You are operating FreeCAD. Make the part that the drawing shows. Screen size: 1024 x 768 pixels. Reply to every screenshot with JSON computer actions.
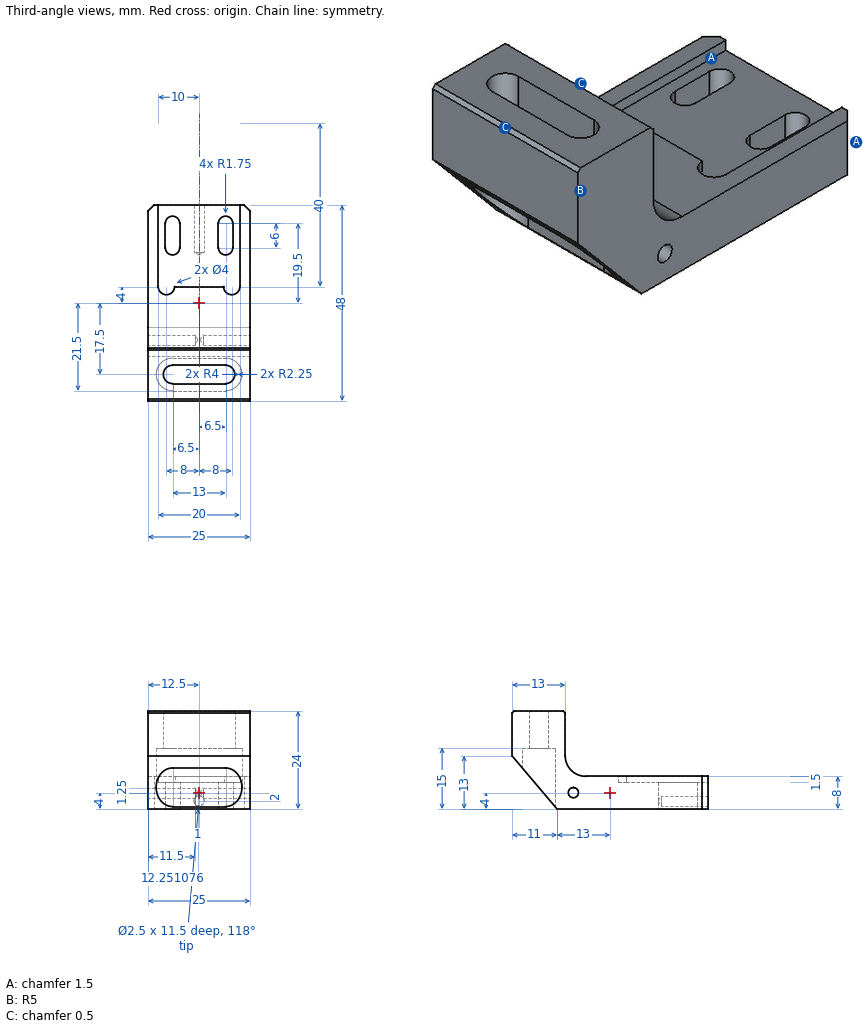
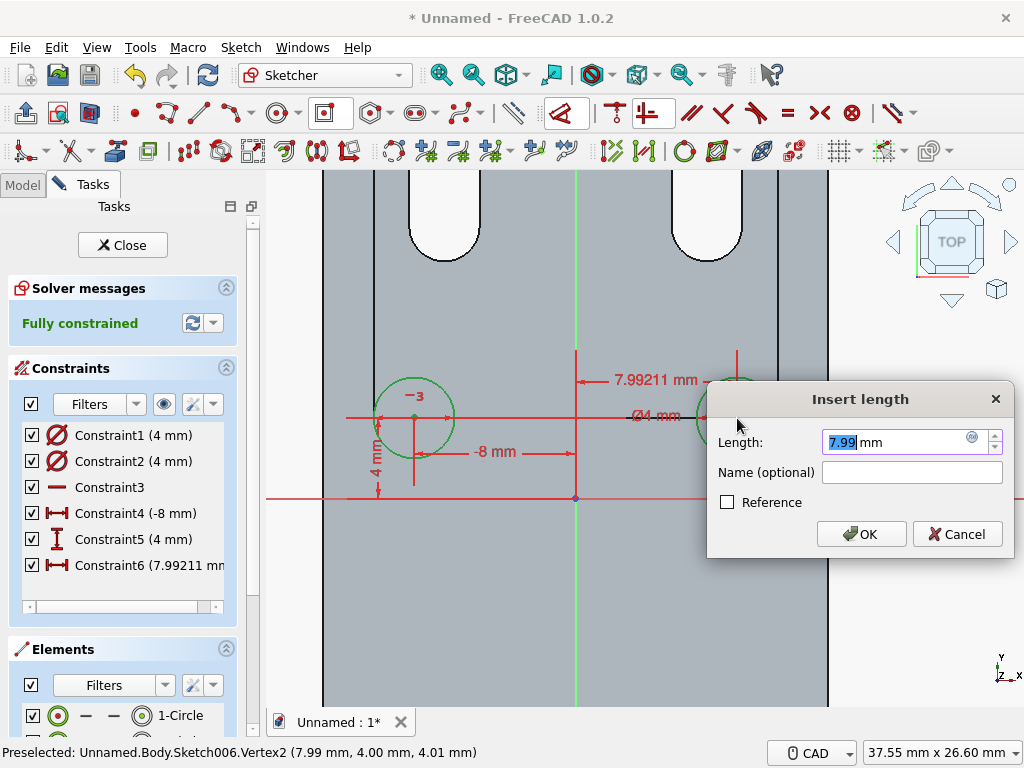
{"action": "type", "text": "8"}
{"action": "key", "text": "Return"}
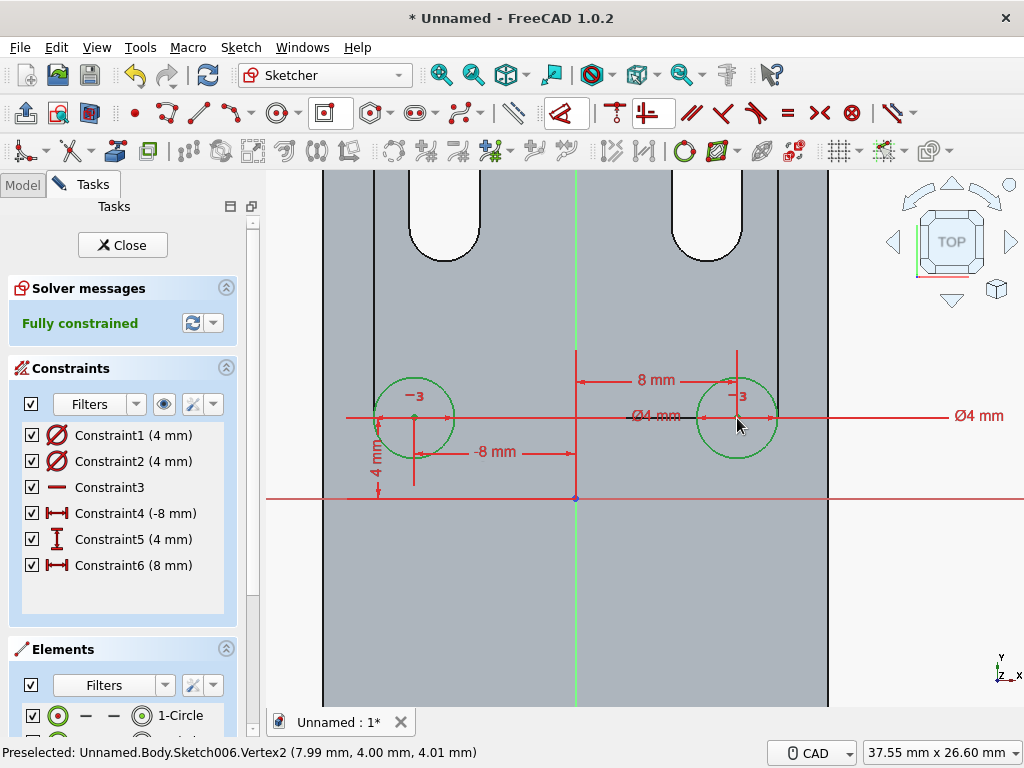
{"action": "left_click", "coordinate": [123, 245]}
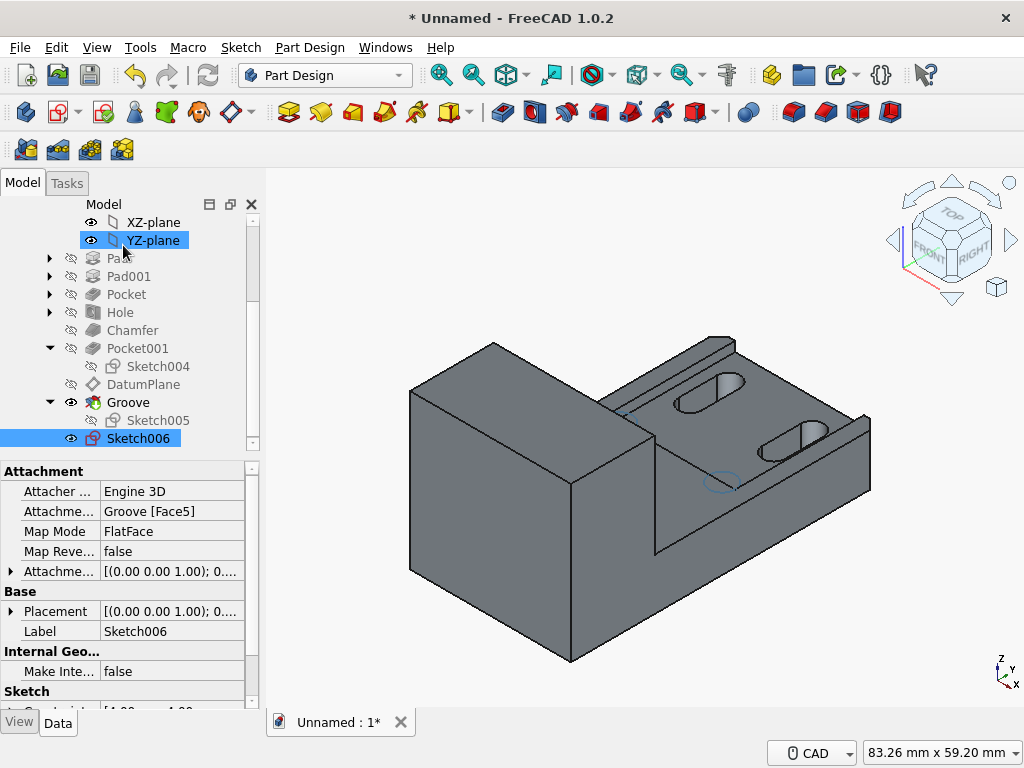
{"action": "left_click", "coordinate": [504, 112]}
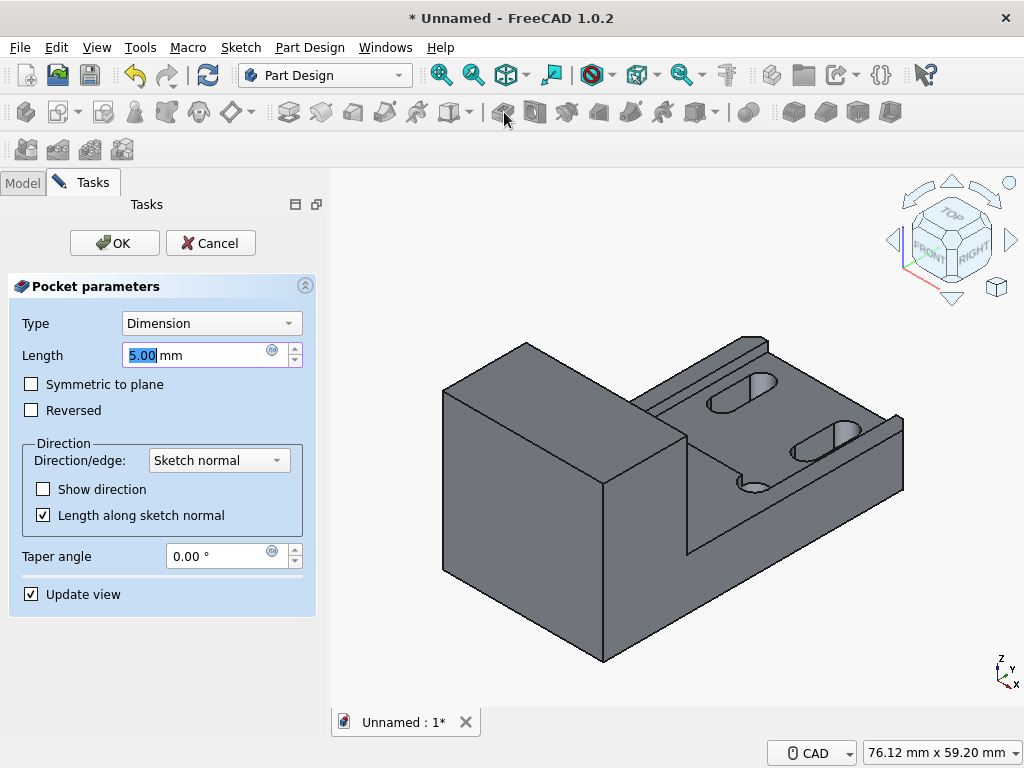
{"action": "type", "text": "1.5"}
{"action": "key", "text": "Tab"}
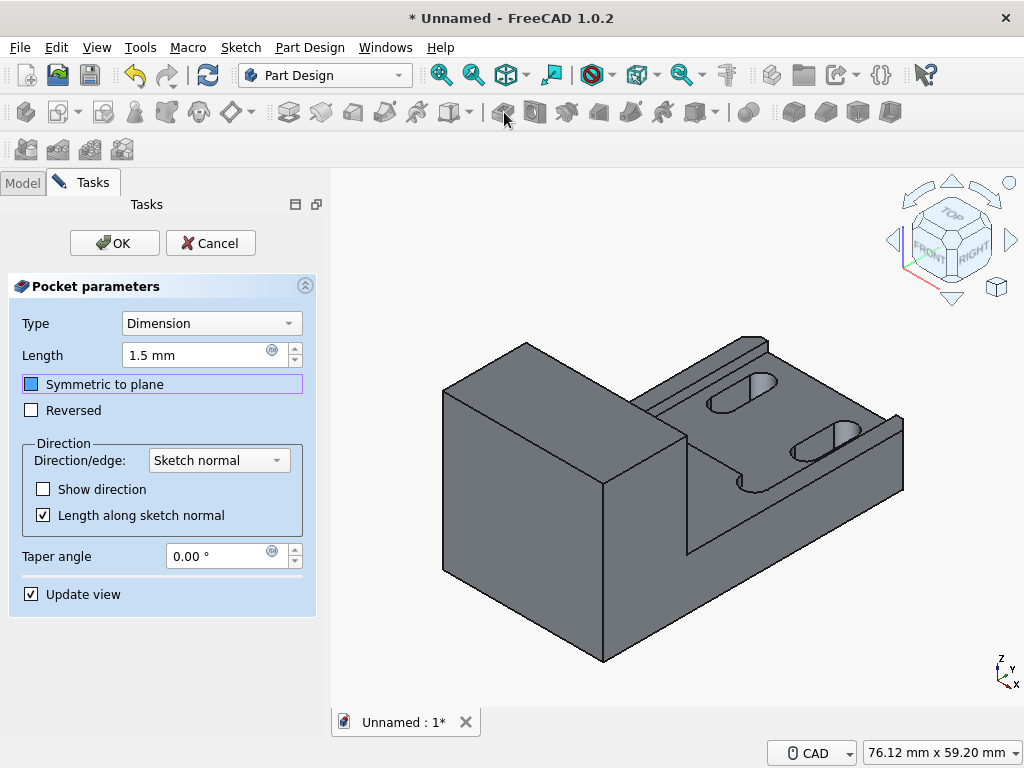
{"action": "left_click", "coordinate": [115, 243]}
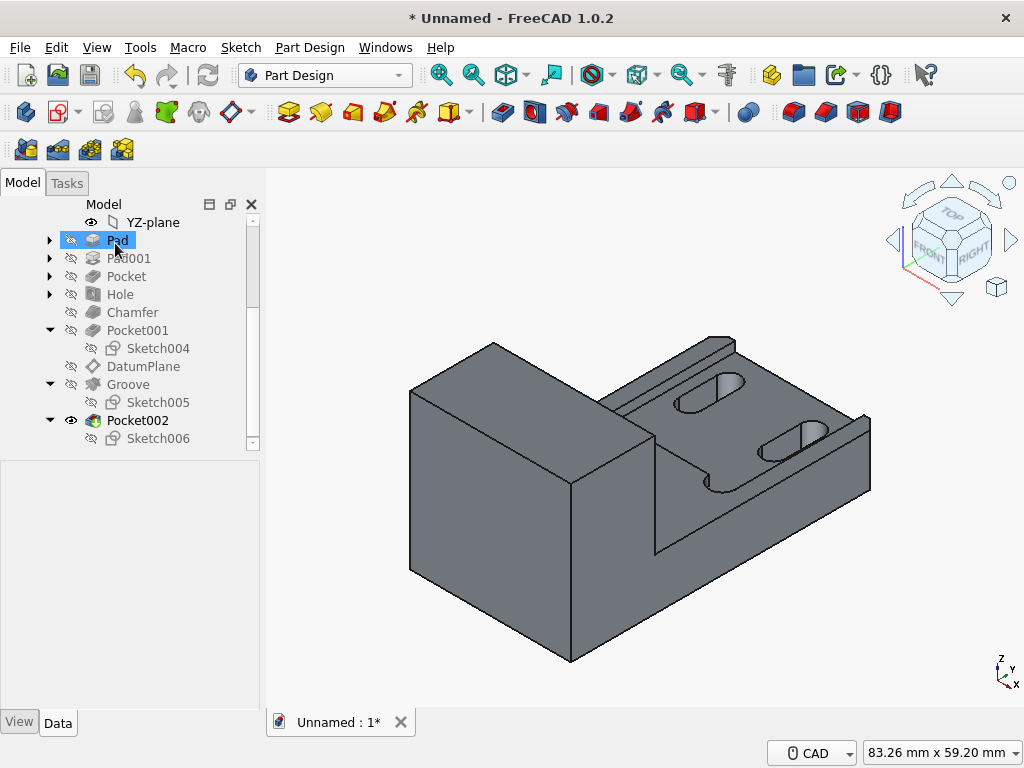
{"action": "key", "text": "5"}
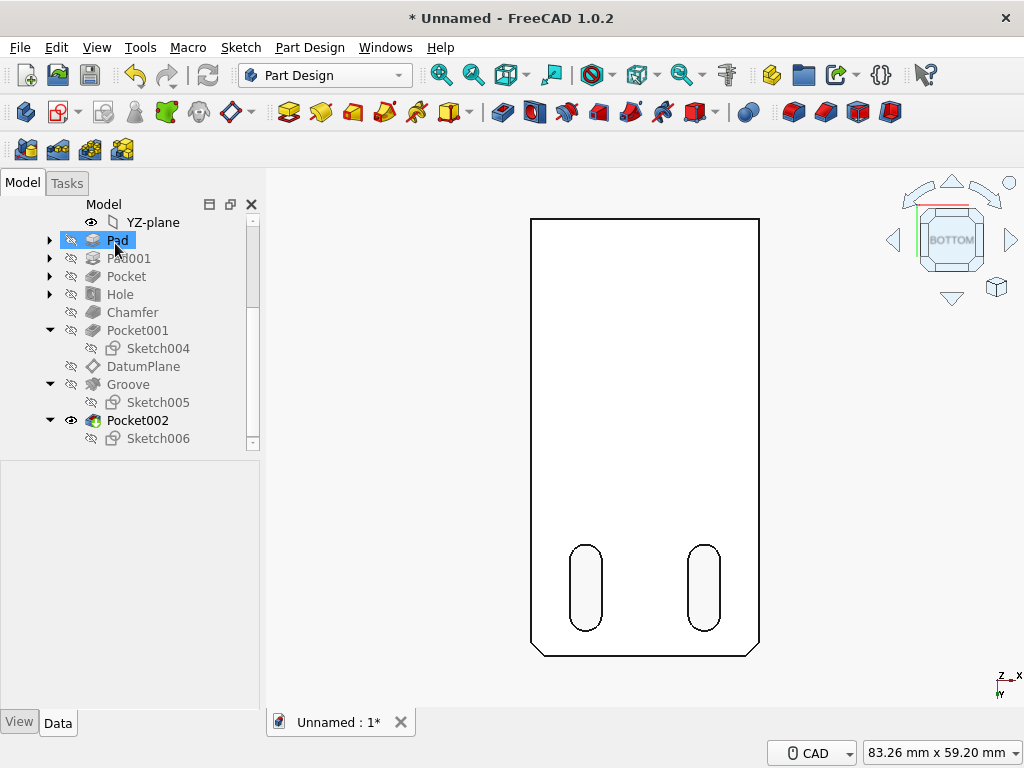
{"action": "left_click", "coordinate": [645, 437]}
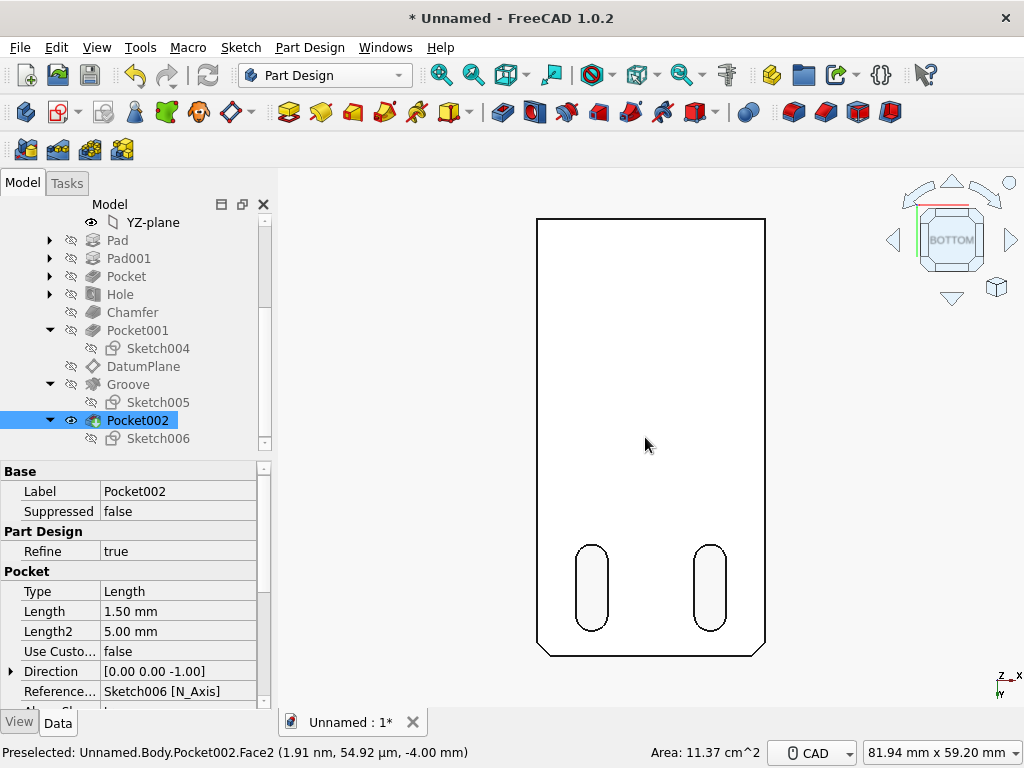
{"action": "left_click", "coordinate": [58, 112]}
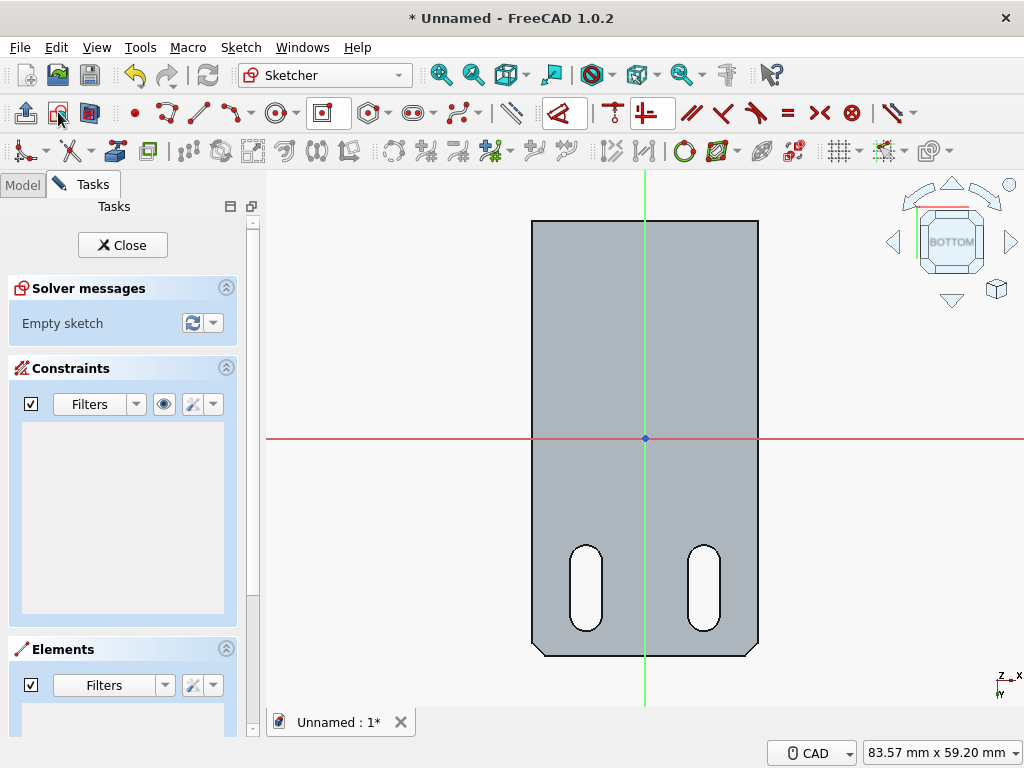
{"action": "scroll", "coordinate": [728, 240], "scroll_direction": "up", "scroll_amount": 3}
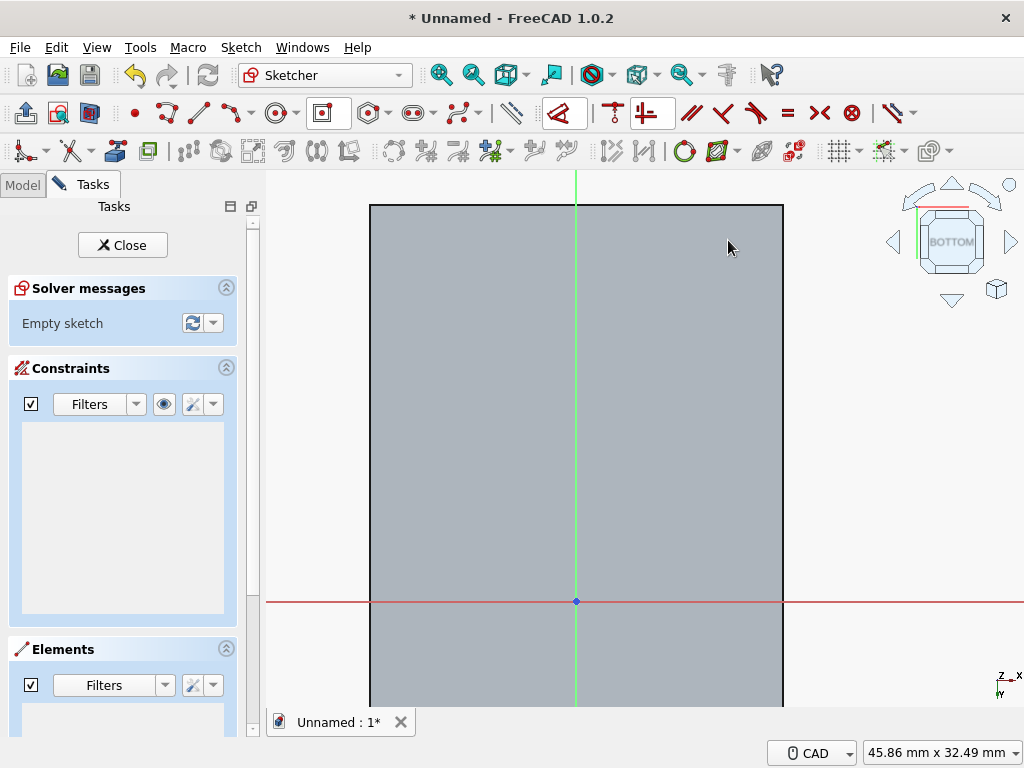
{"action": "left_click", "coordinate": [414, 114]}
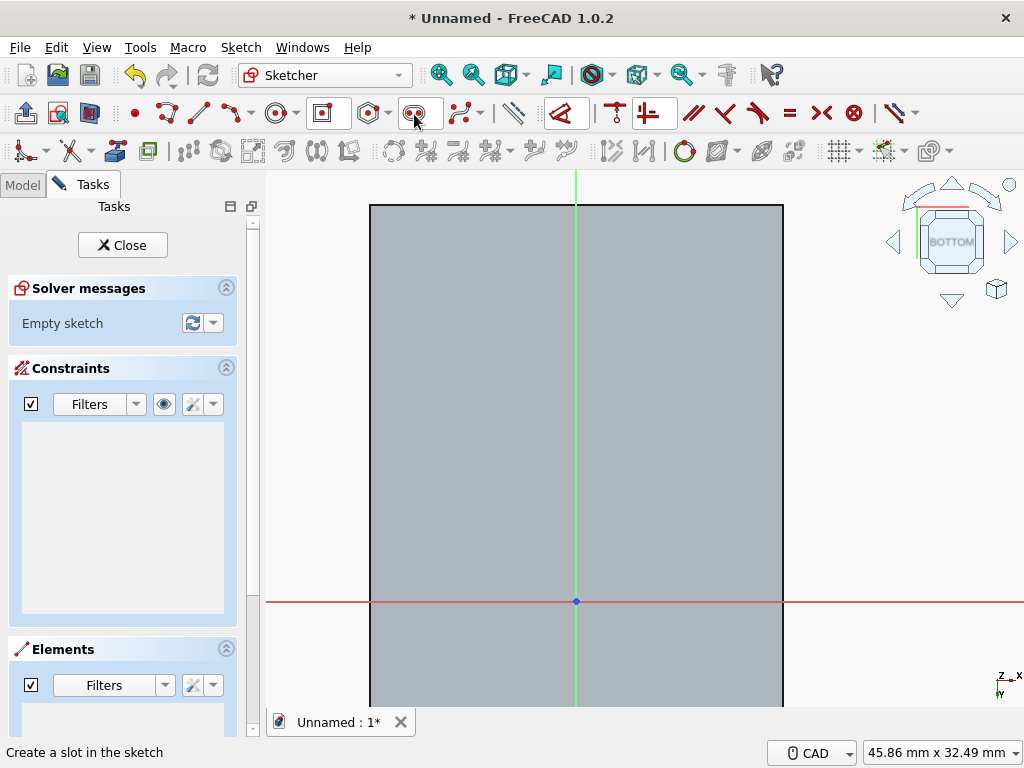
{"action": "left_click", "coordinate": [469, 312]}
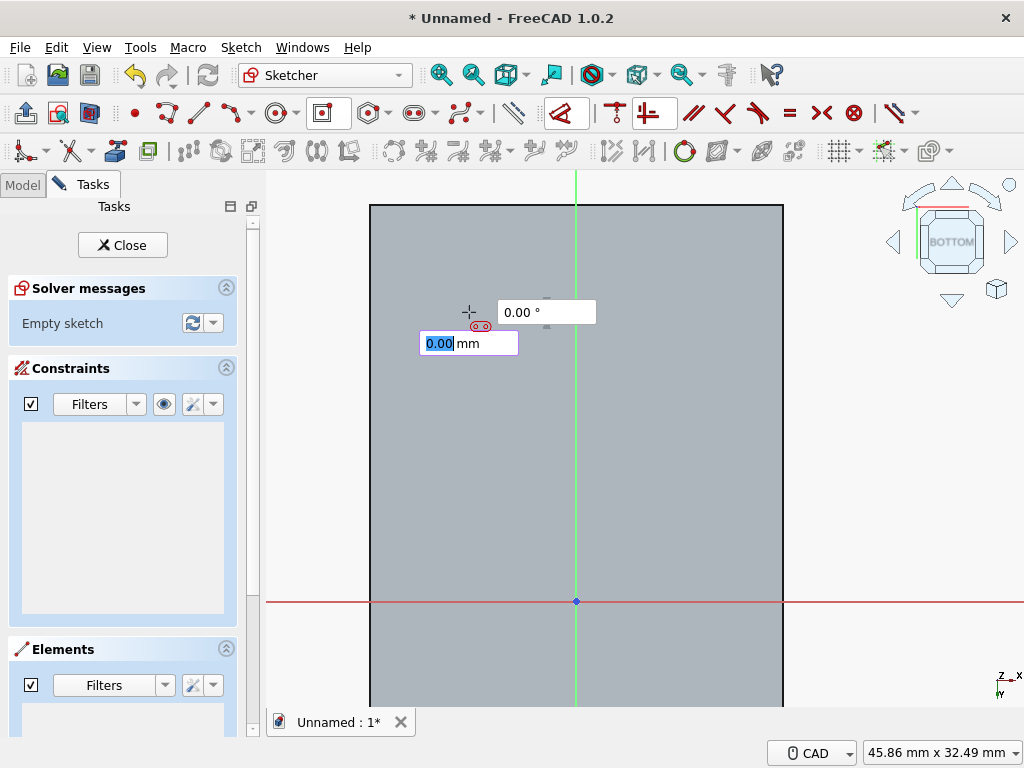
{"action": "left_click", "coordinate": [684, 312]}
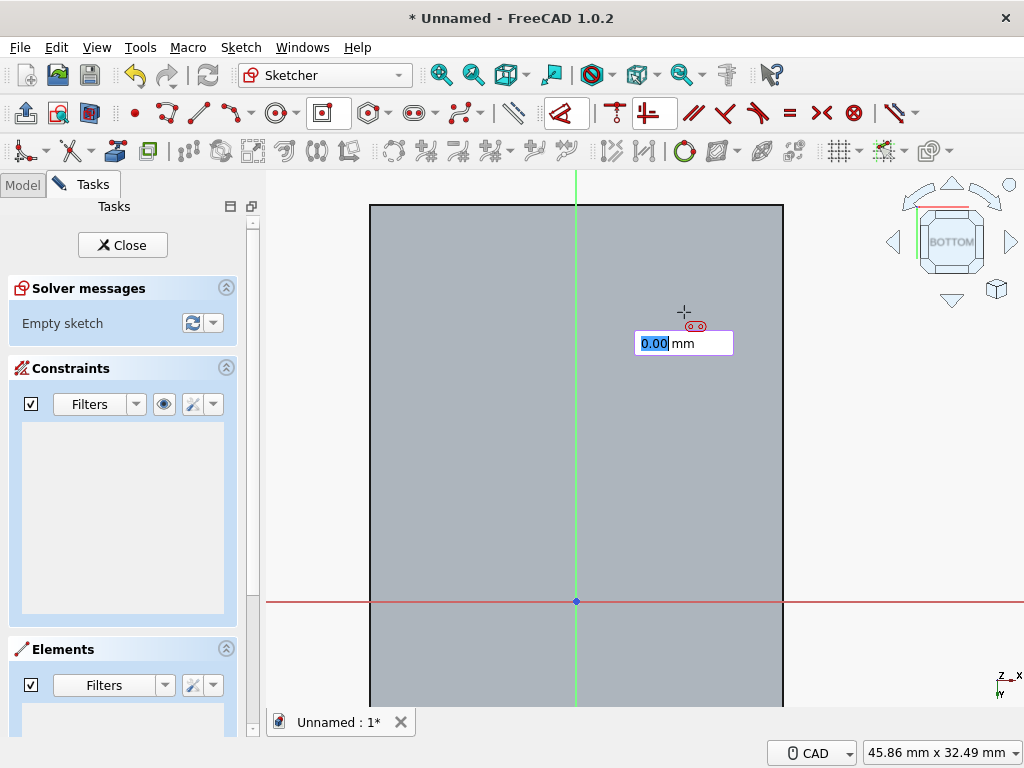
{"action": "left_click", "coordinate": [544, 350]}
{"action": "key", "text": "Escape"}